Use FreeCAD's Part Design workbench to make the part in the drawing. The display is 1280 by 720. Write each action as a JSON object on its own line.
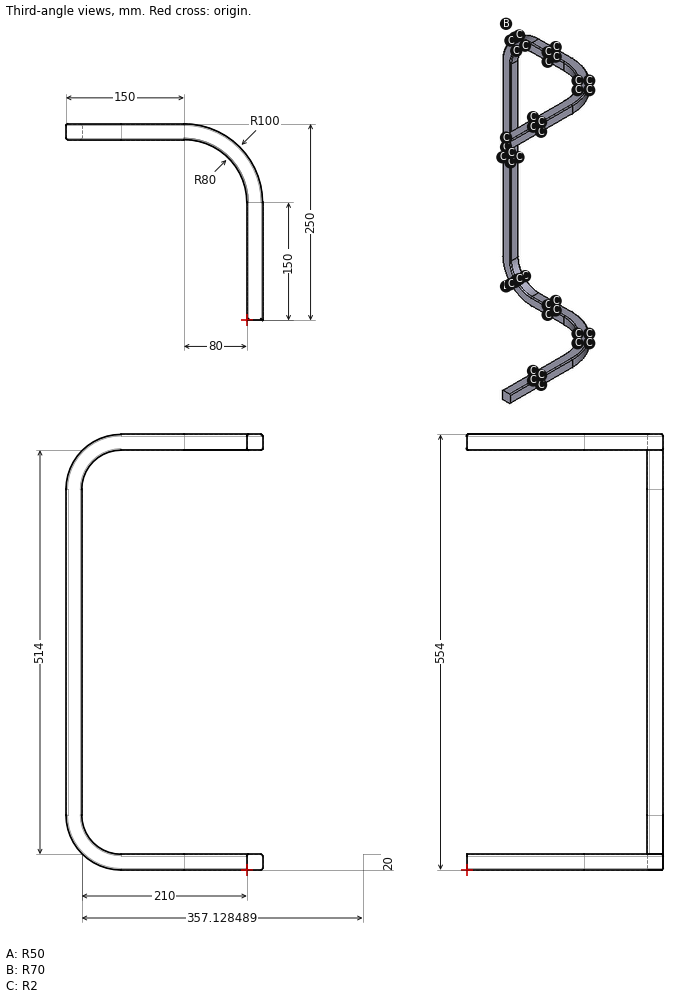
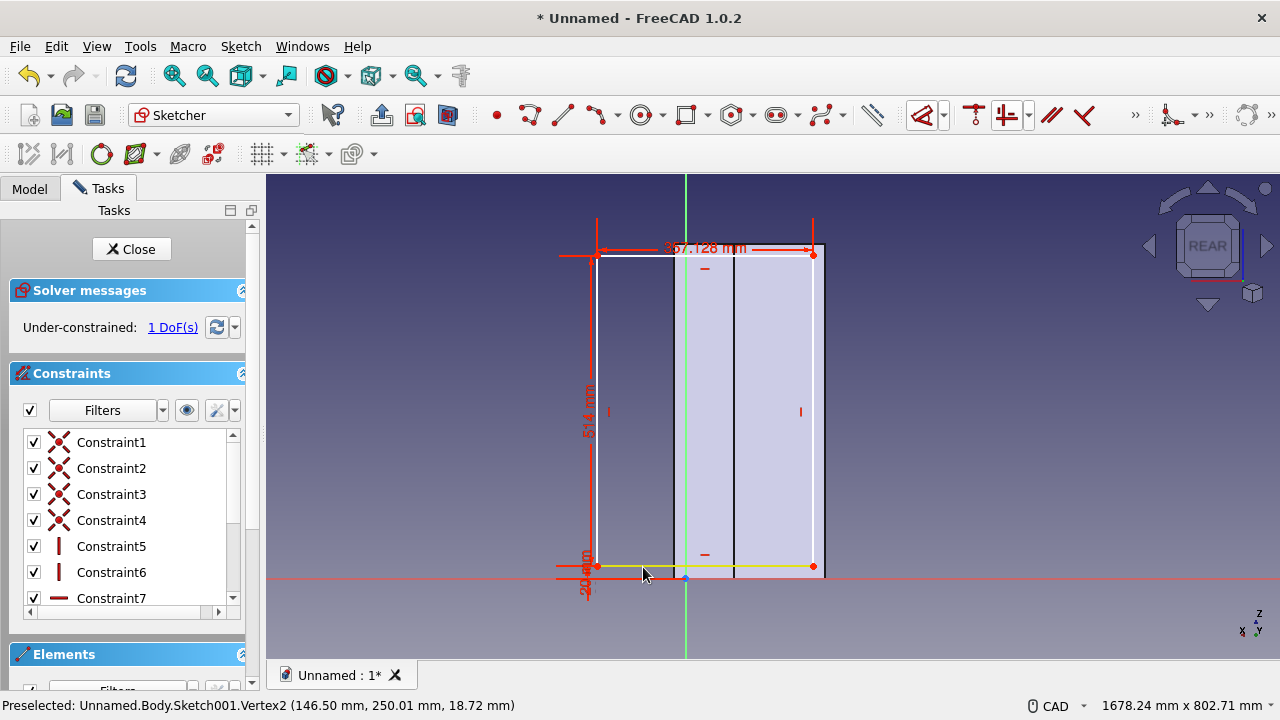
{"action": "left_click", "coordinate": [813, 566]}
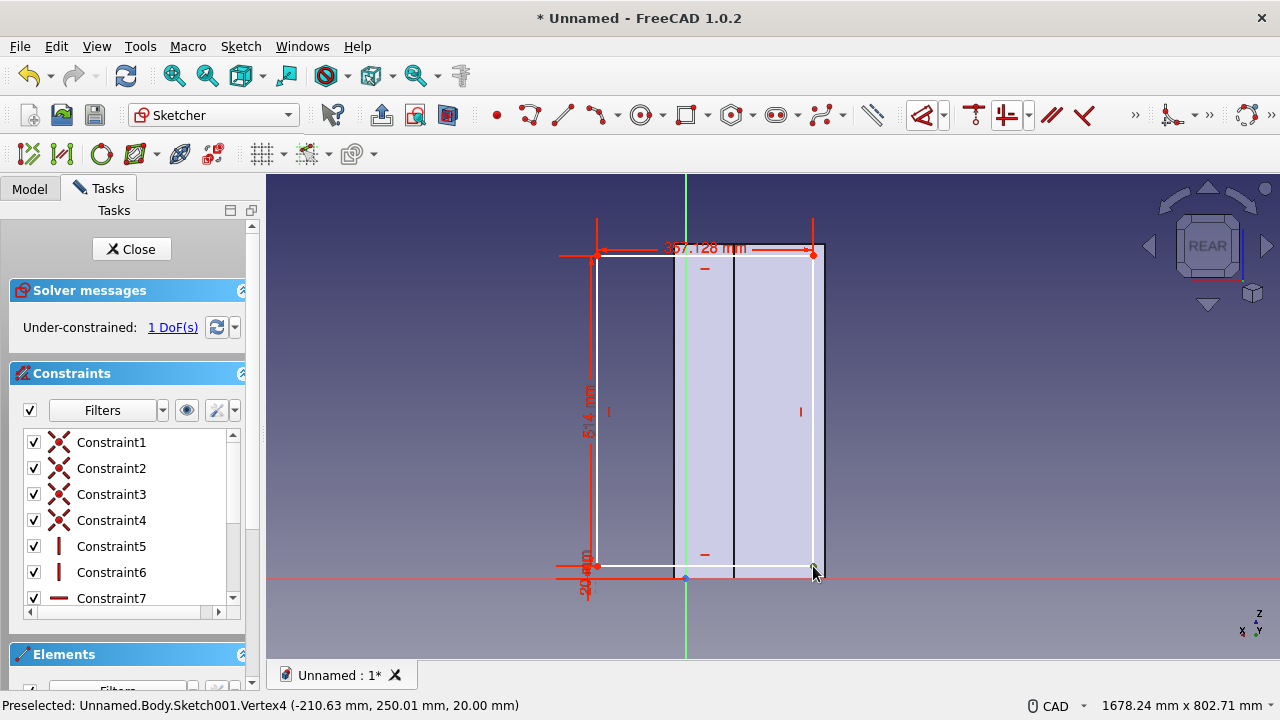
{"action": "left_click", "coordinate": [944, 116]}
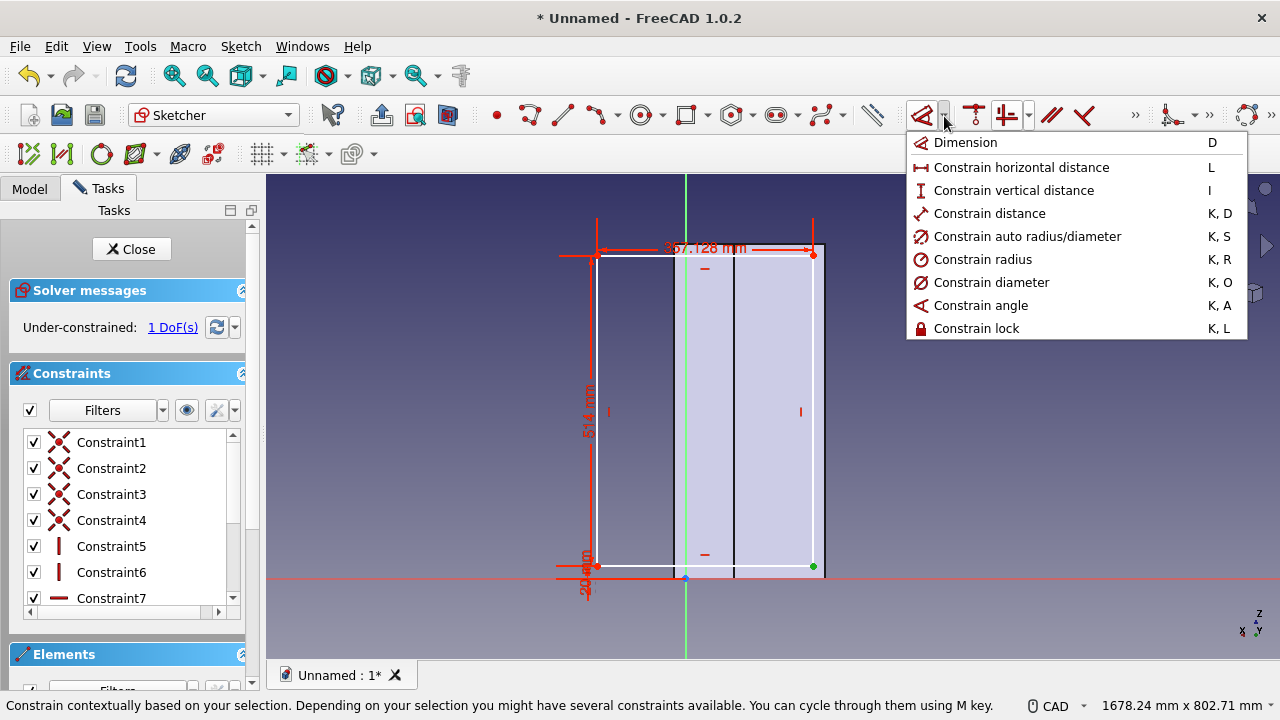
{"action": "left_click", "coordinate": [1077, 168]}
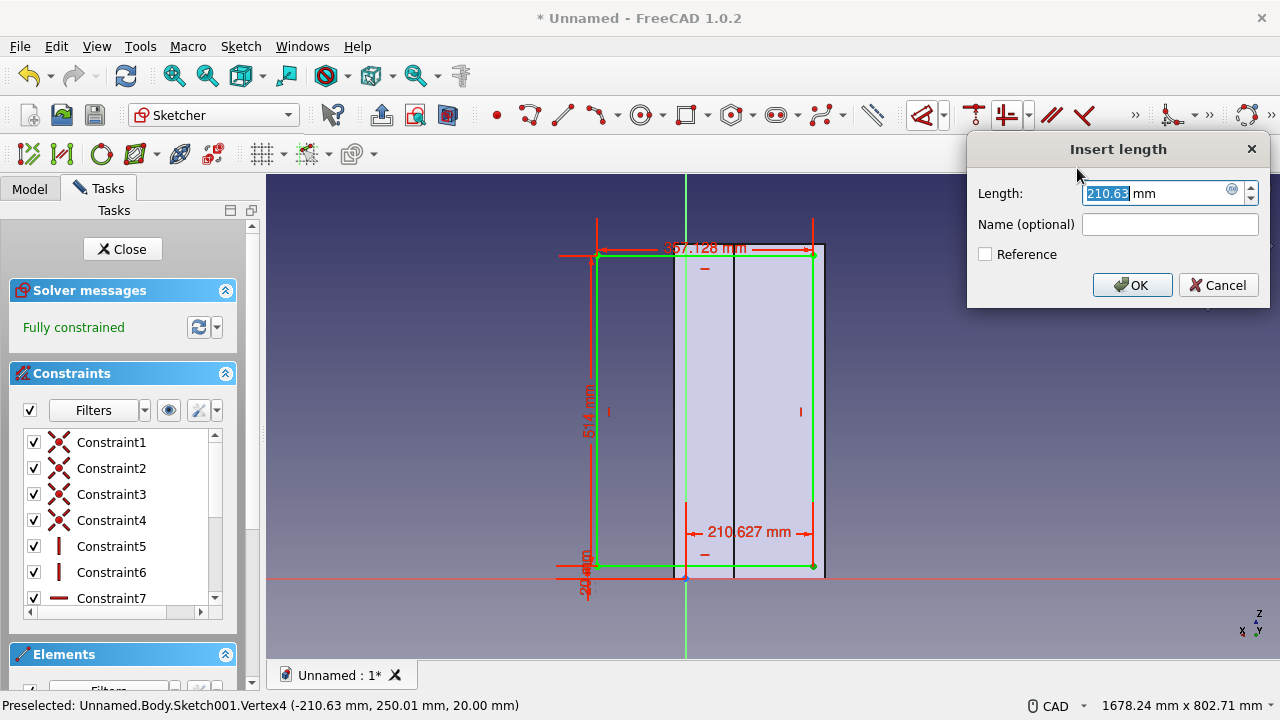
{"action": "type", "text": "210"}
{"action": "key", "text": "Return"}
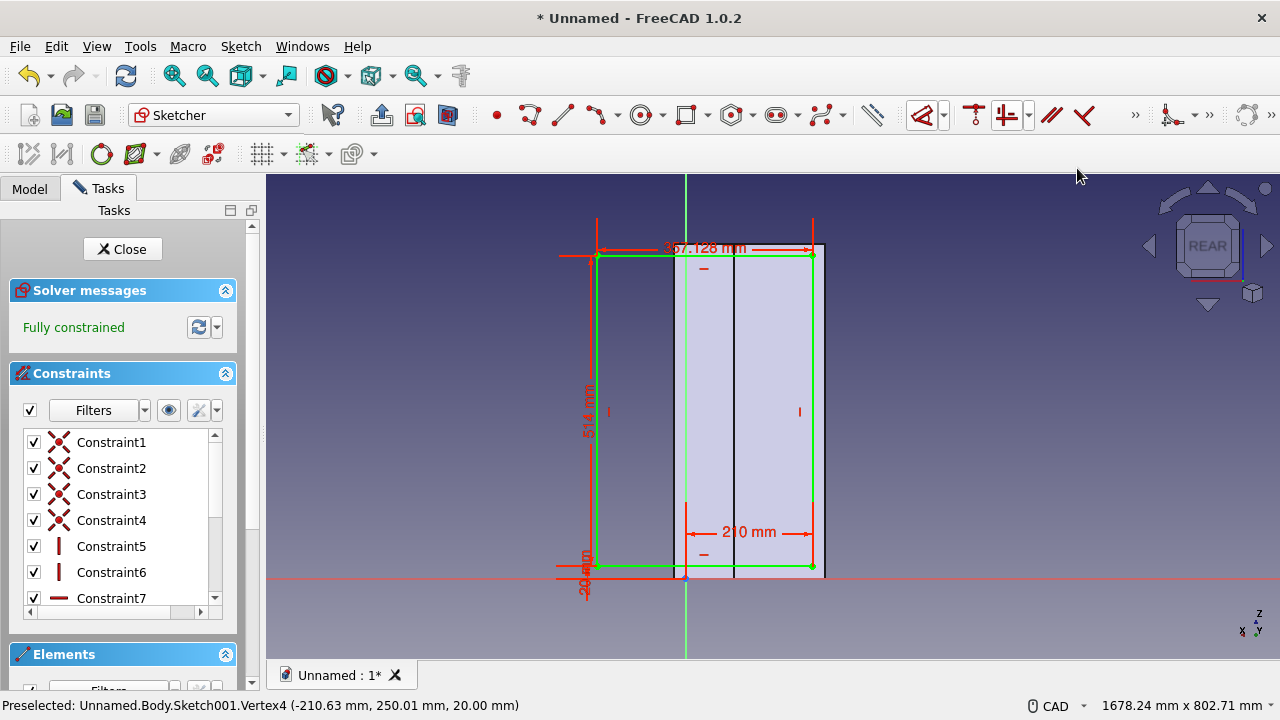
{"action": "left_click", "coordinate": [123, 249]}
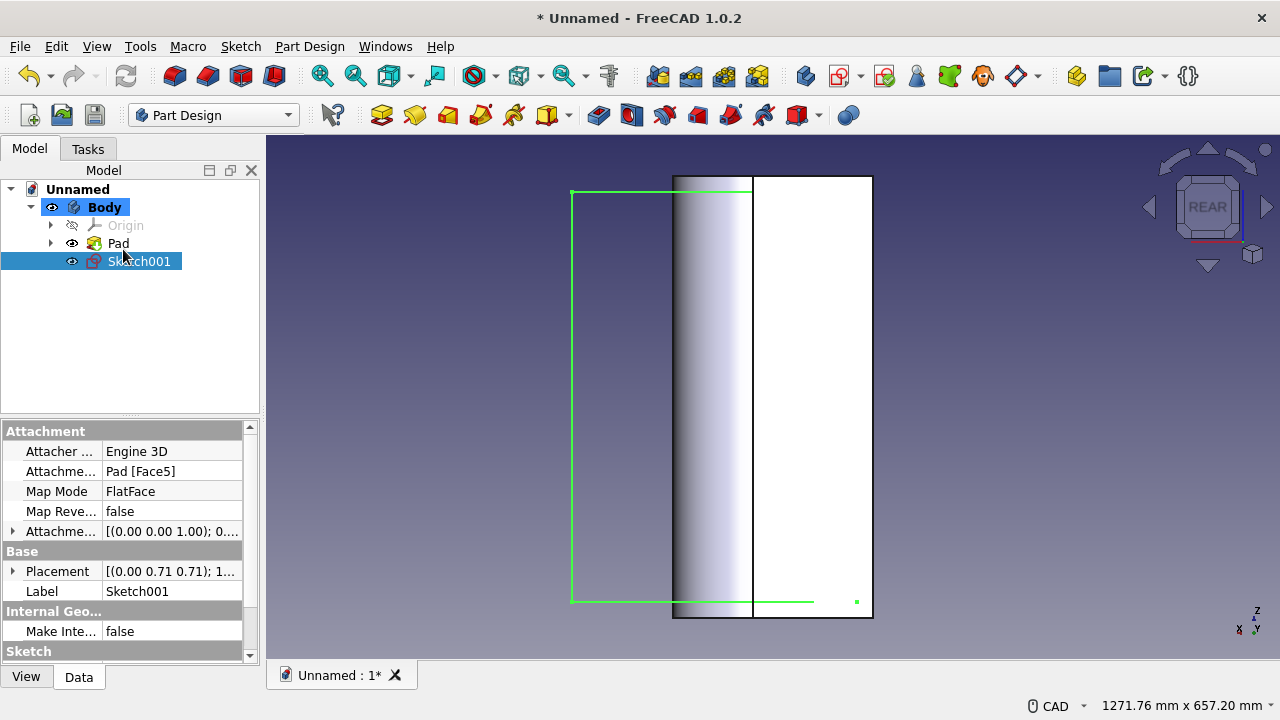
{"action": "left_click", "coordinate": [599, 116]}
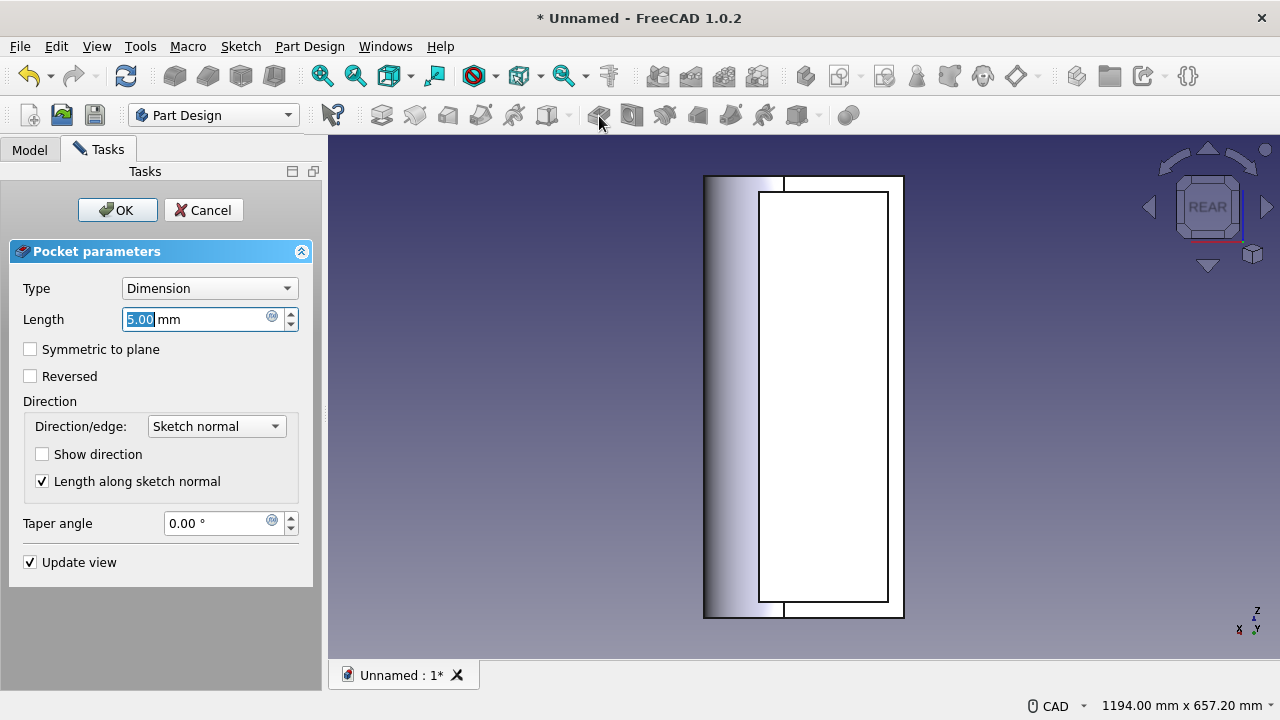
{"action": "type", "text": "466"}
{"action": "key", "text": "Tab"}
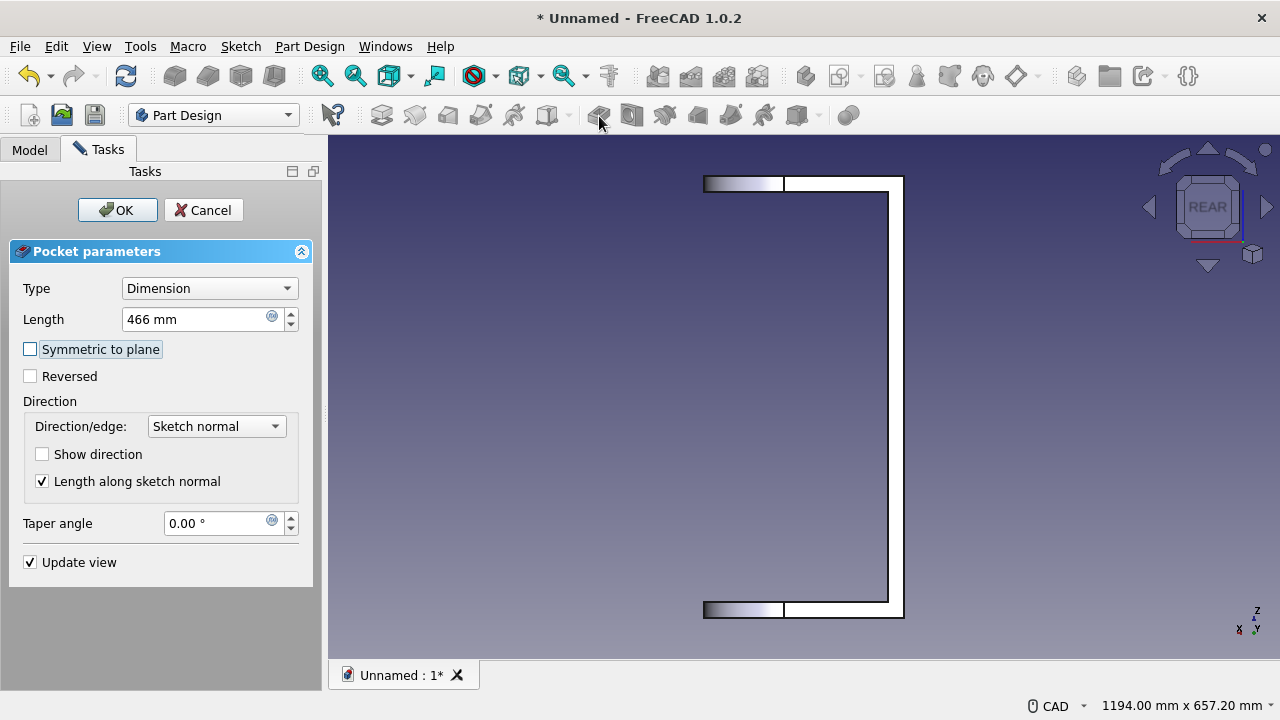
{"action": "left_click", "coordinate": [118, 210]}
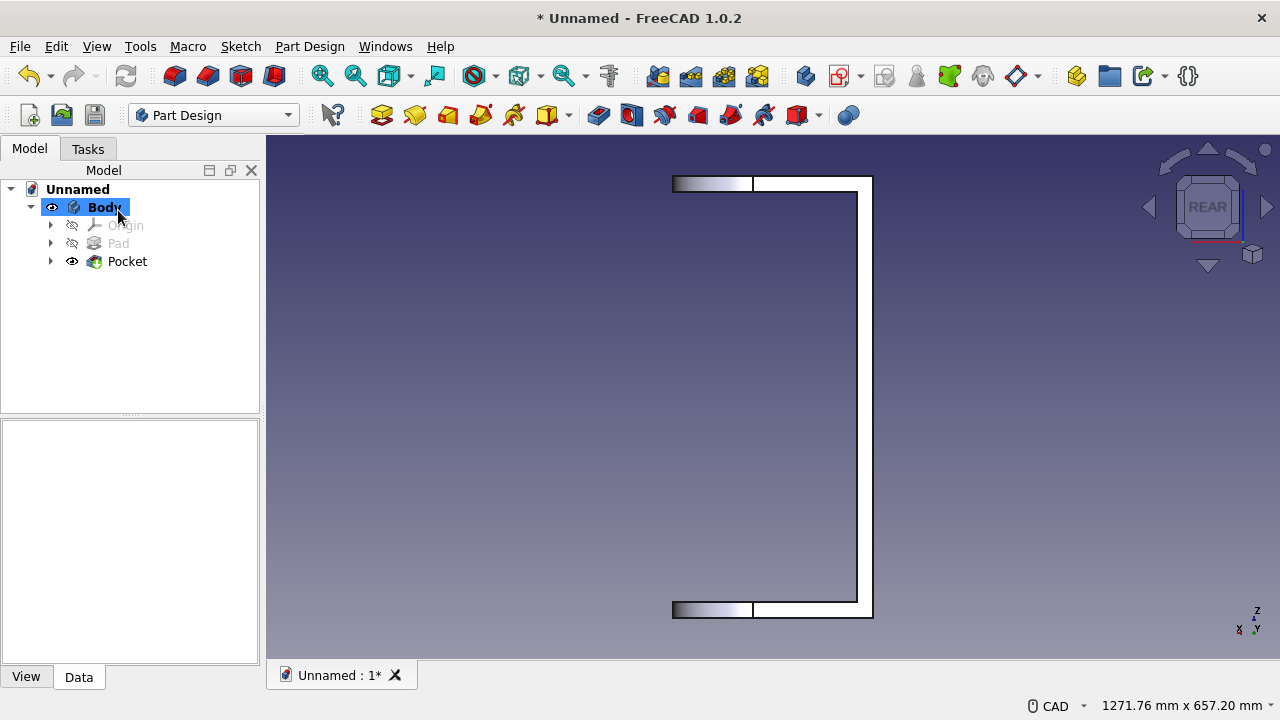
{"action": "scroll", "coordinate": [857, 191], "scroll_direction": "up", "scroll_amount": 5}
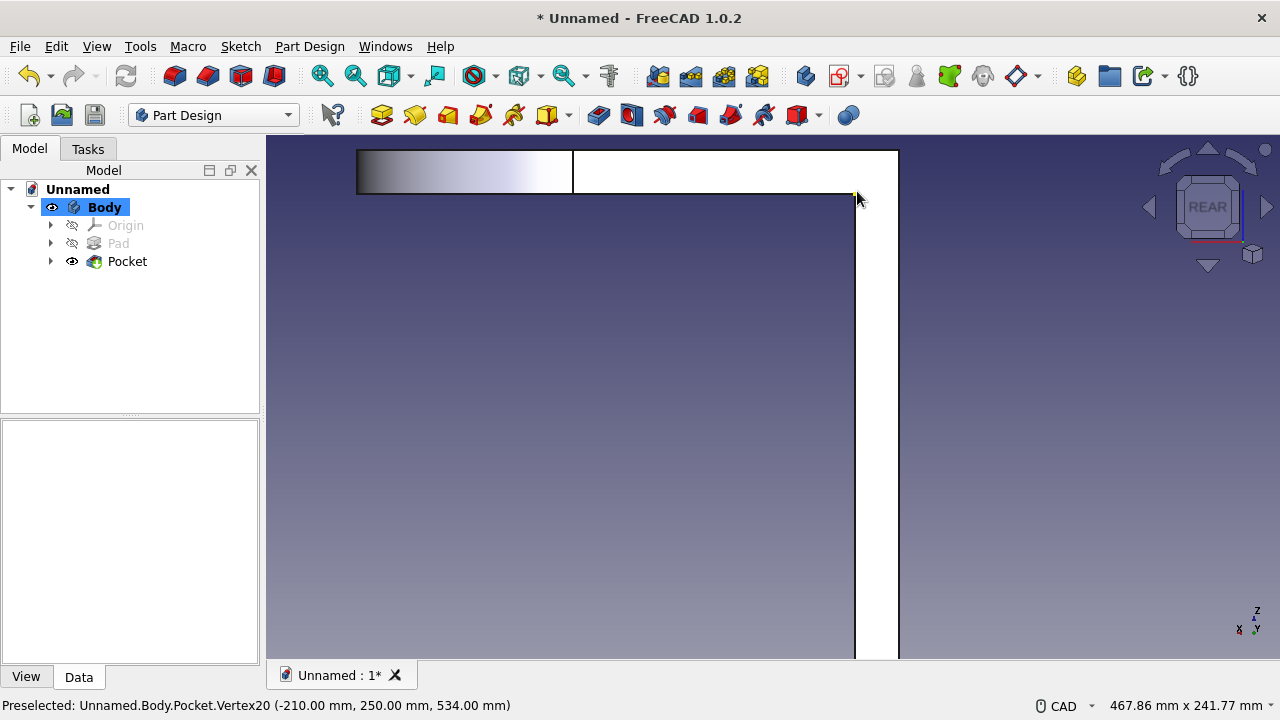
{"action": "left_click", "coordinate": [323, 76]}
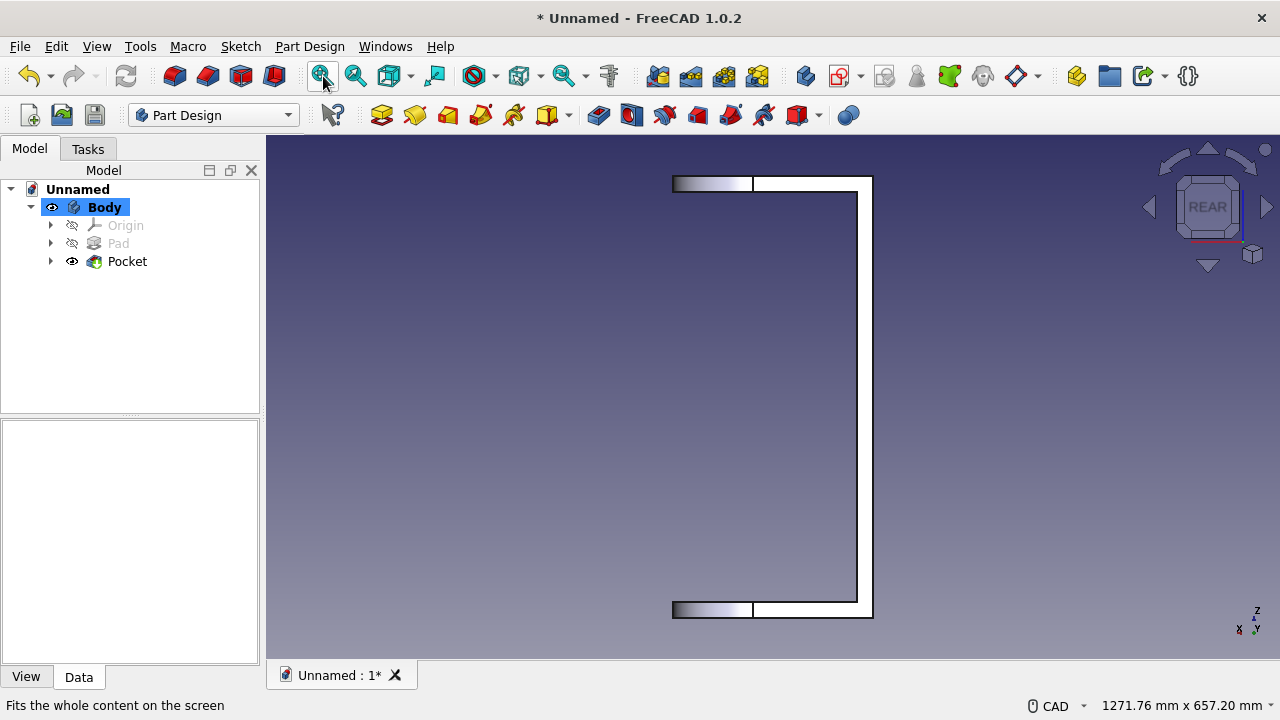
{"action": "key", "text": "0"}